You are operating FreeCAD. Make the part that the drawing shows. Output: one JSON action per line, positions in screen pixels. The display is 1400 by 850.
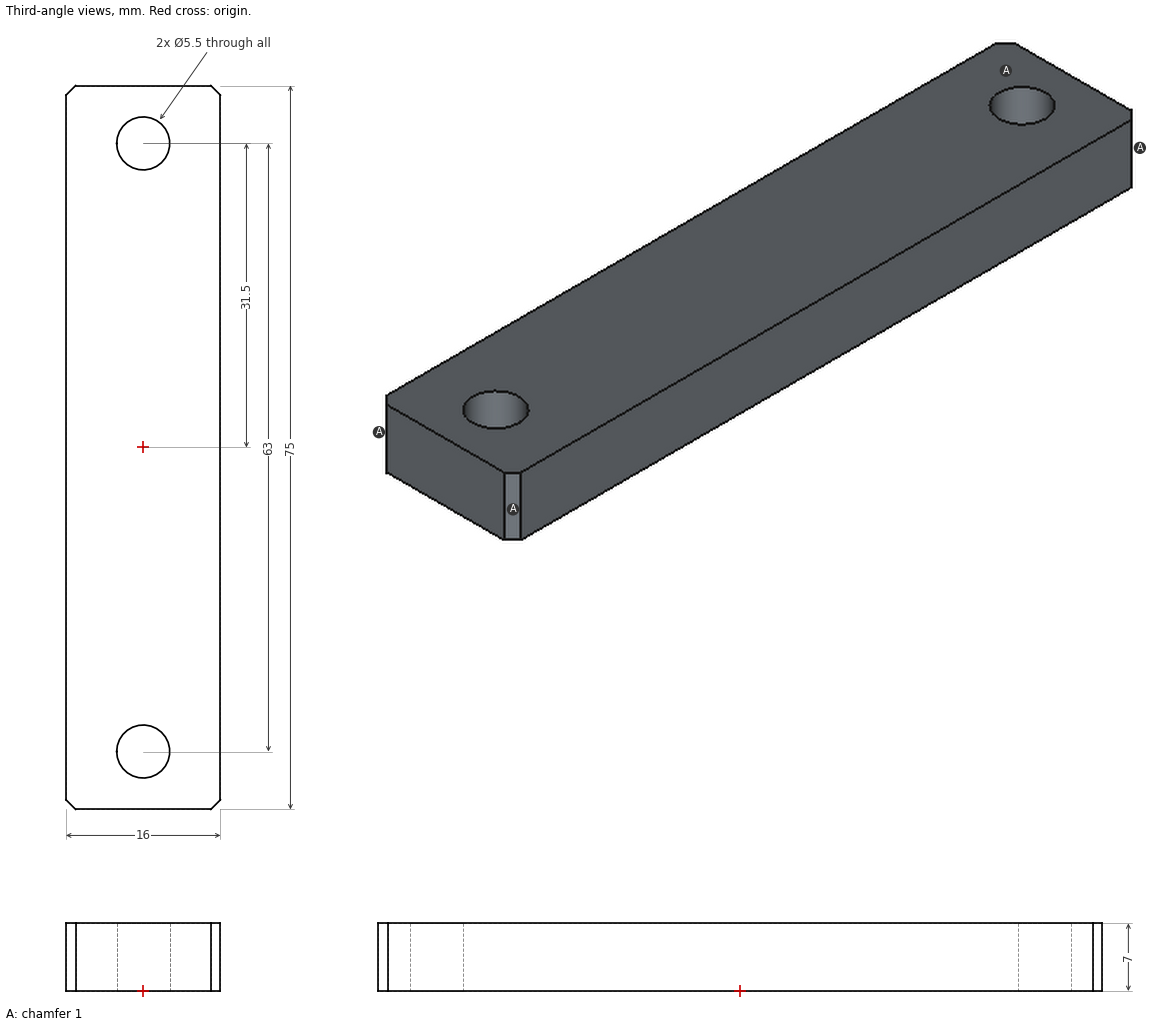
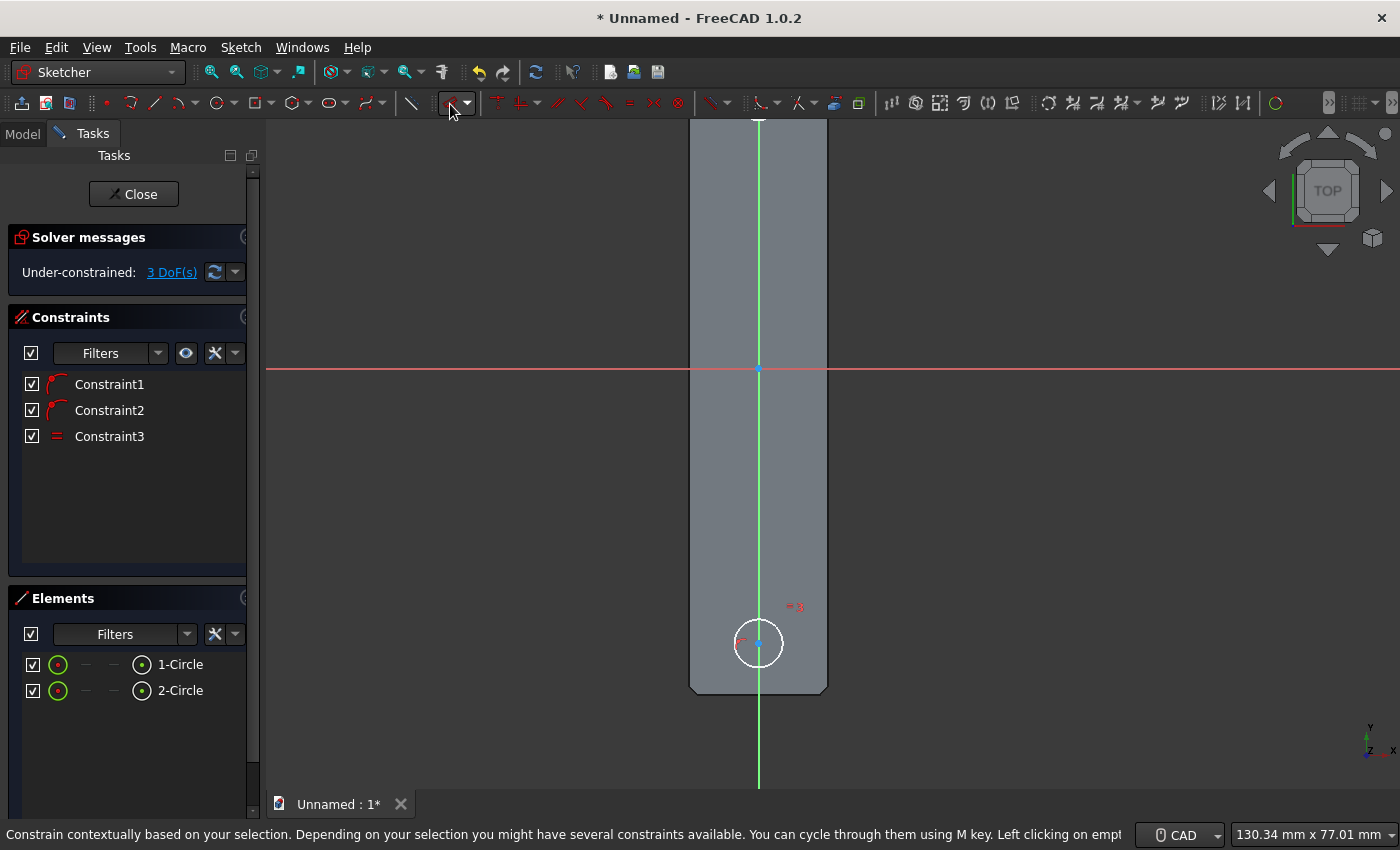
{"action": "scroll", "coordinate": [776, 627], "scroll_direction": "down", "scroll_amount": 2}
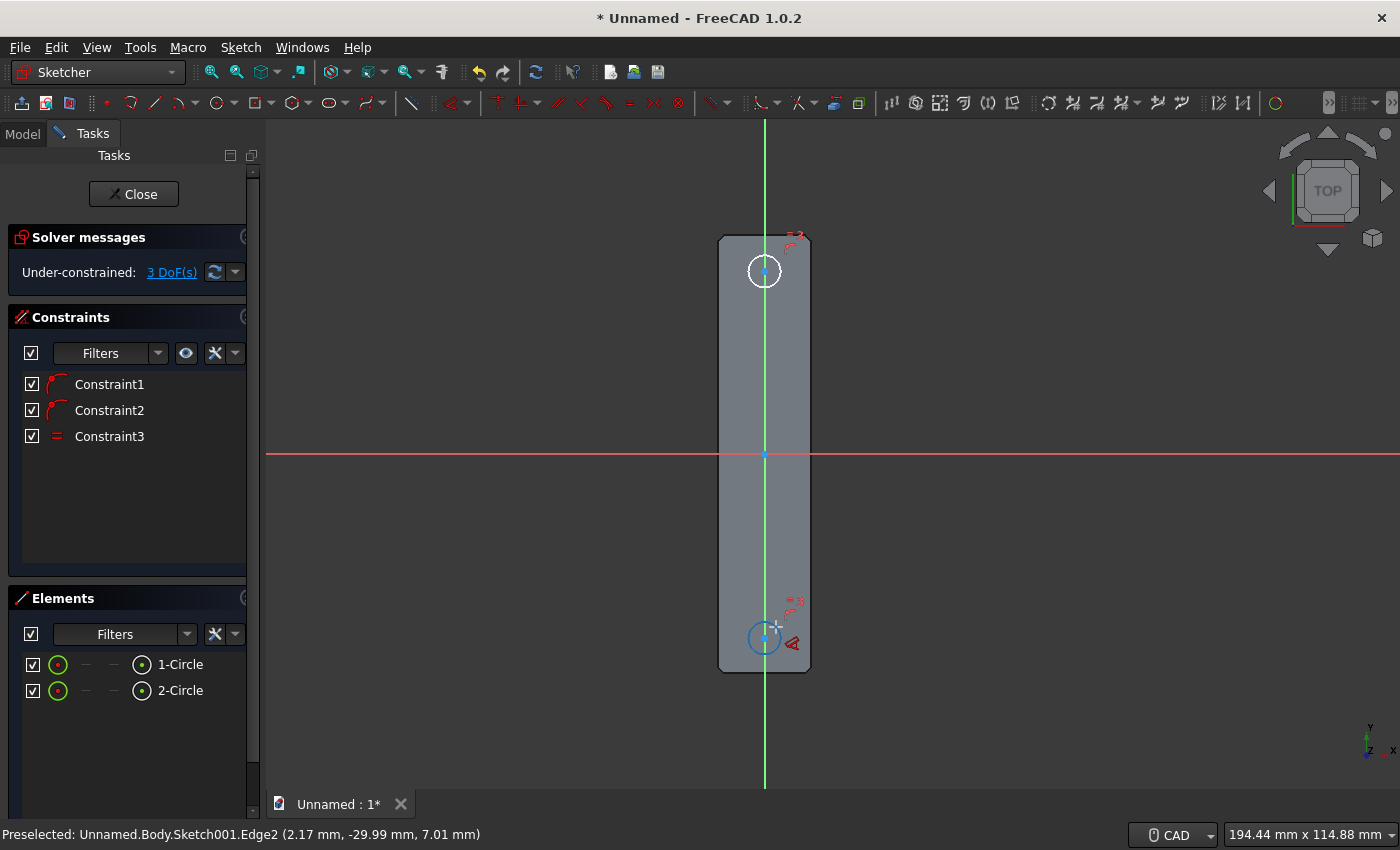
{"action": "scroll", "coordinate": [776, 260], "scroll_direction": "up", "scroll_amount": 2}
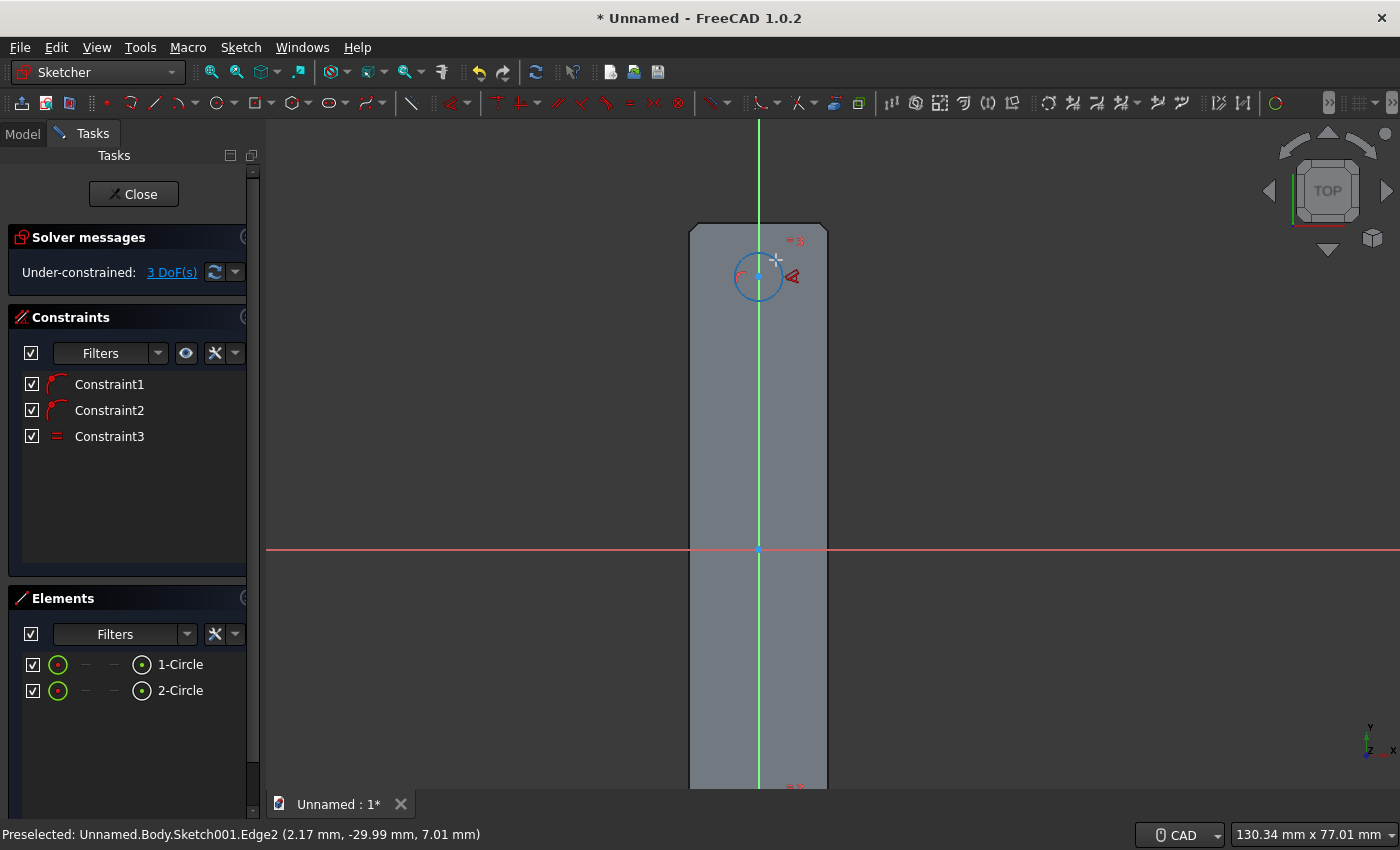
{"action": "left_click", "coordinate": [776, 260]}
{"action": "left_click", "coordinate": [799, 238]}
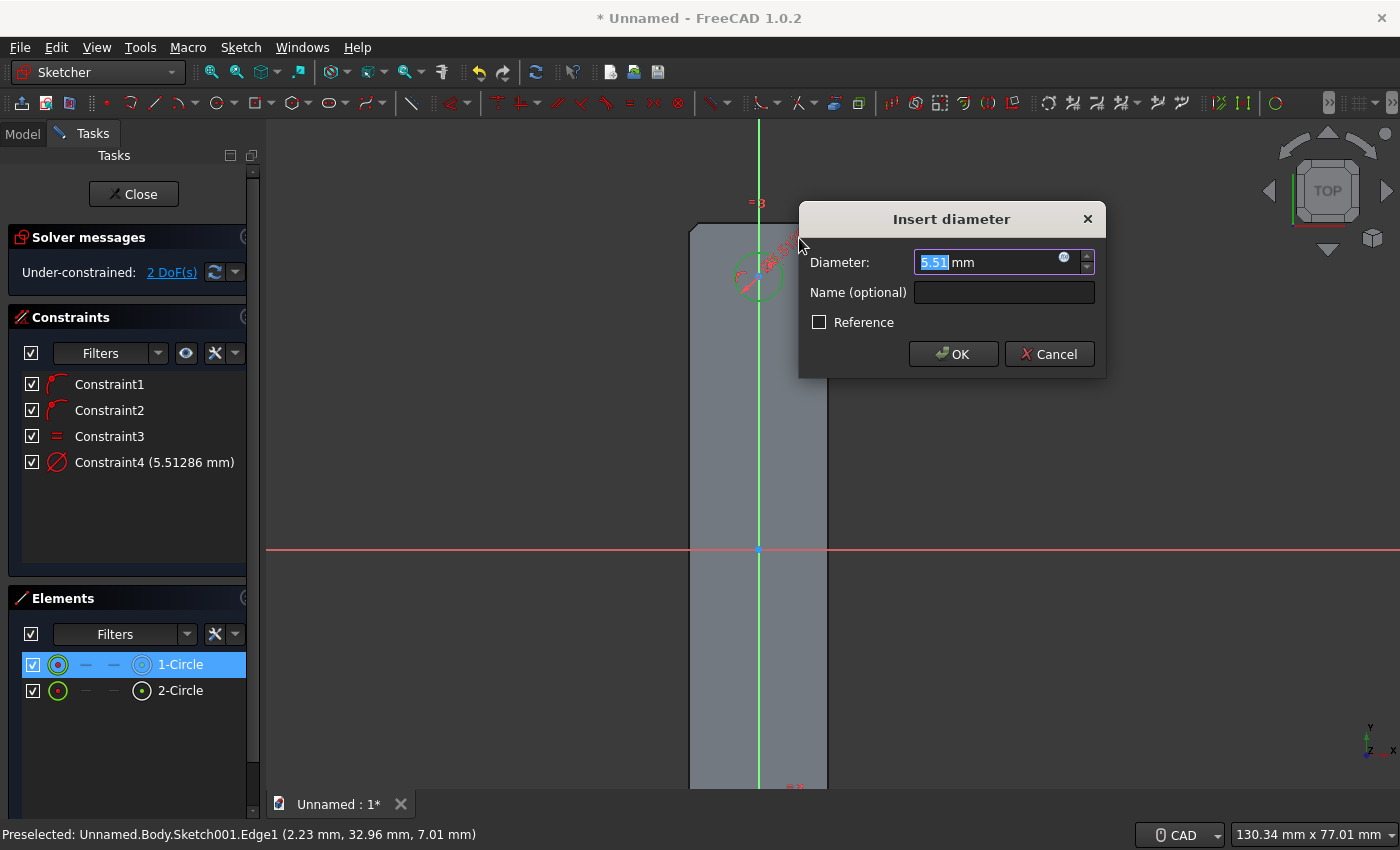
{"action": "type", "text": "5.5"}
{"action": "key", "text": "Return"}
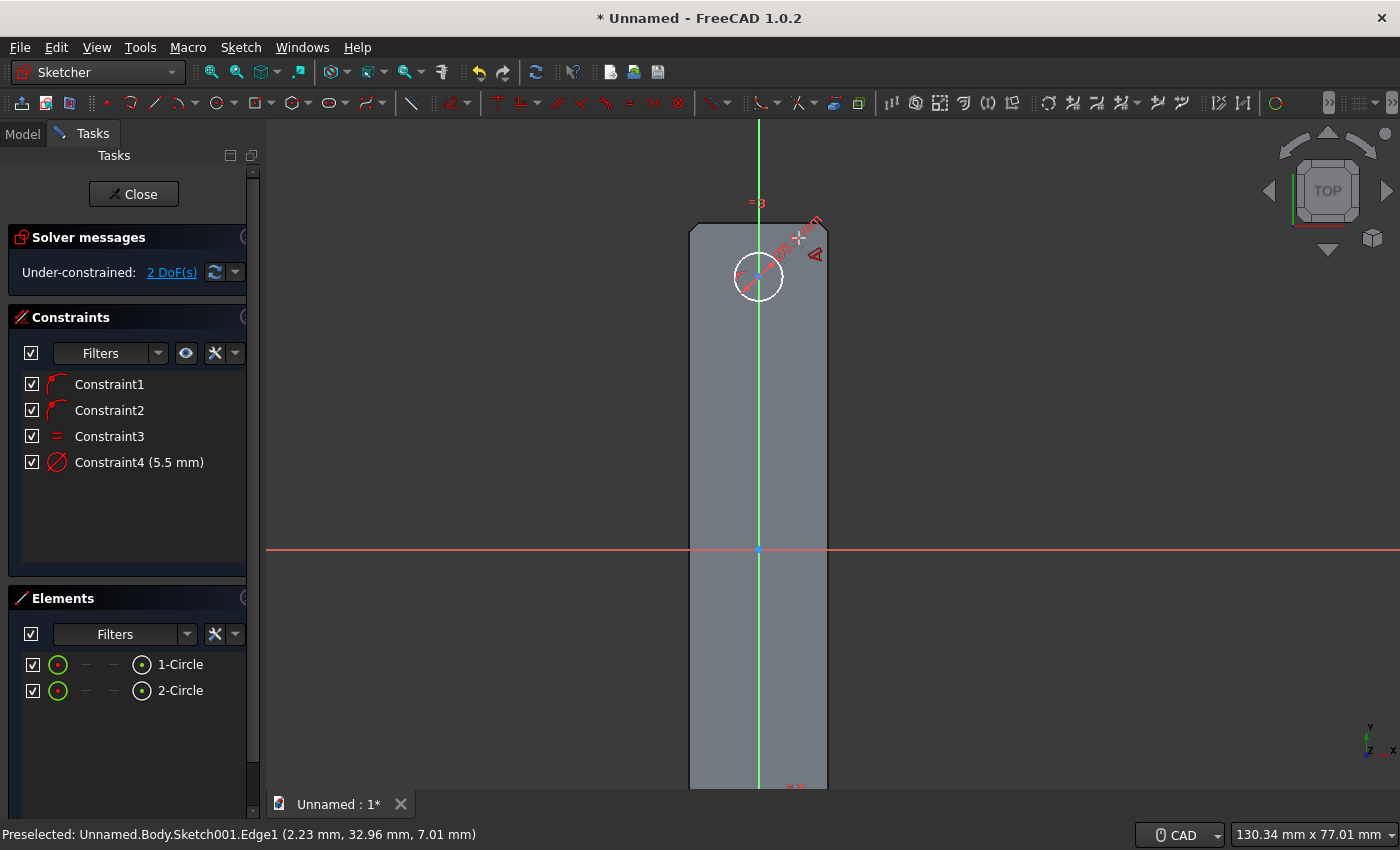
{"action": "left_click", "coordinate": [759, 277]}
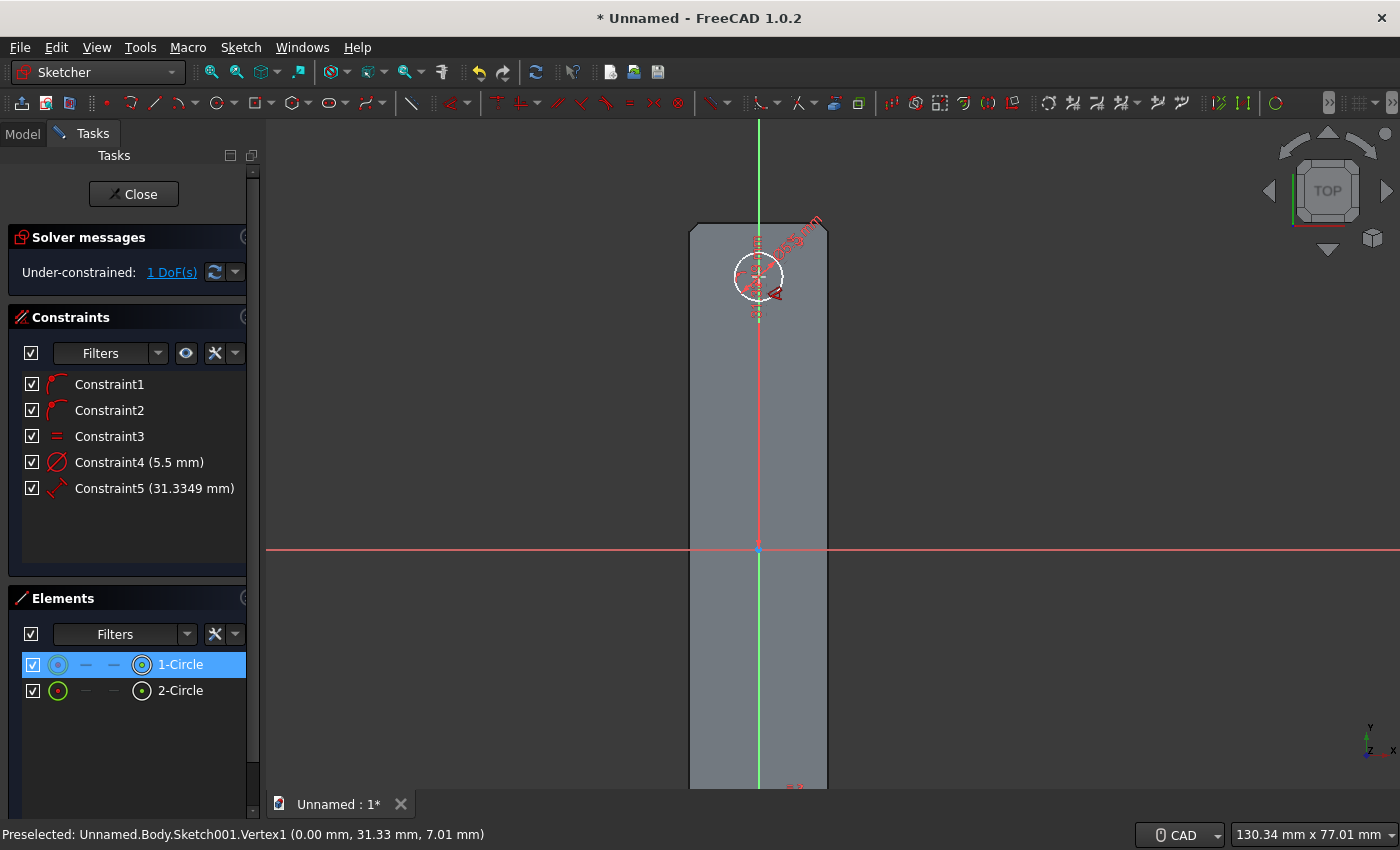
{"action": "scroll", "coordinate": [776, 260], "scroll_direction": "down", "scroll_amount": 2}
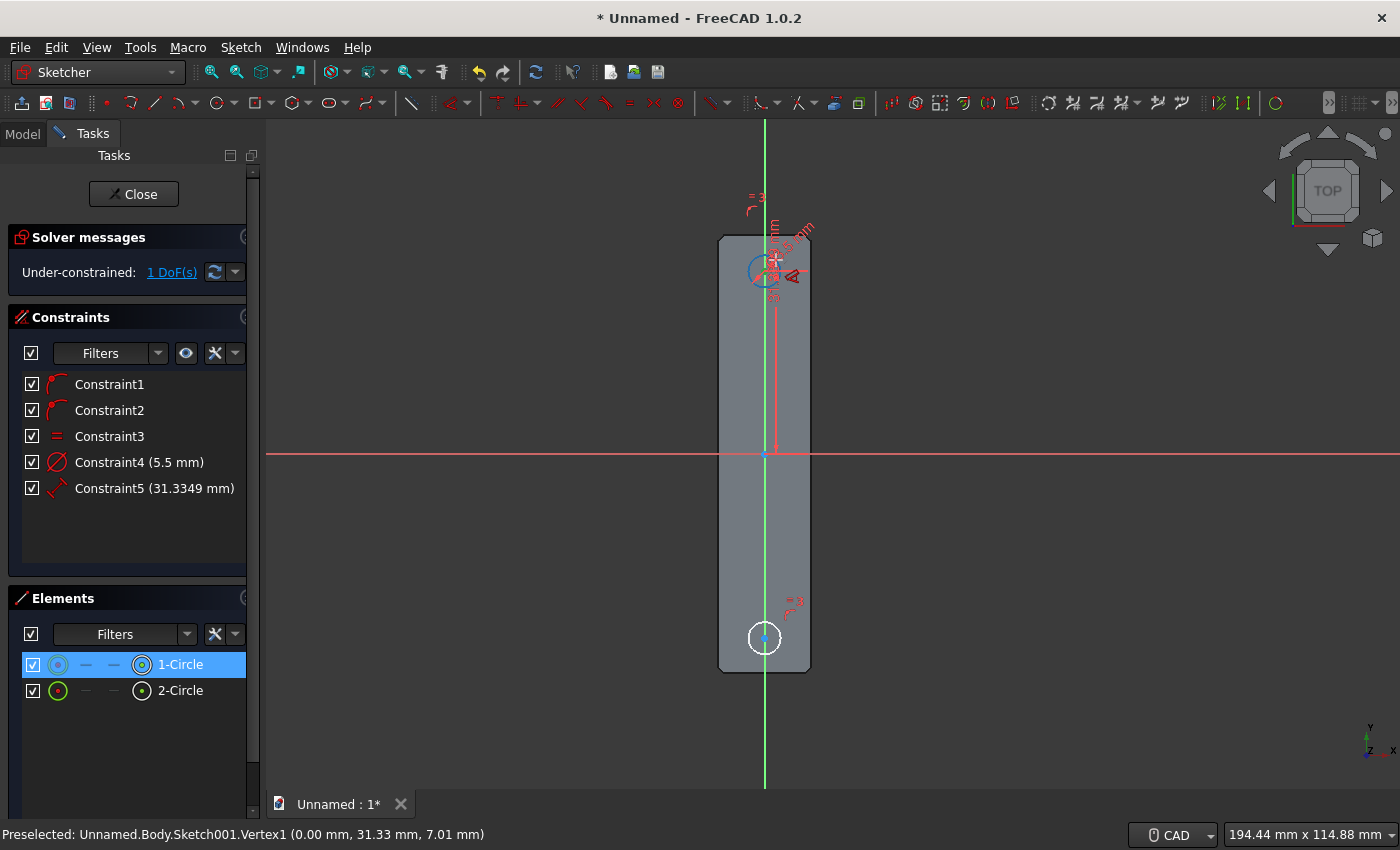
{"action": "left_click", "coordinate": [765, 638]}
{"action": "left_click", "coordinate": [799, 370]}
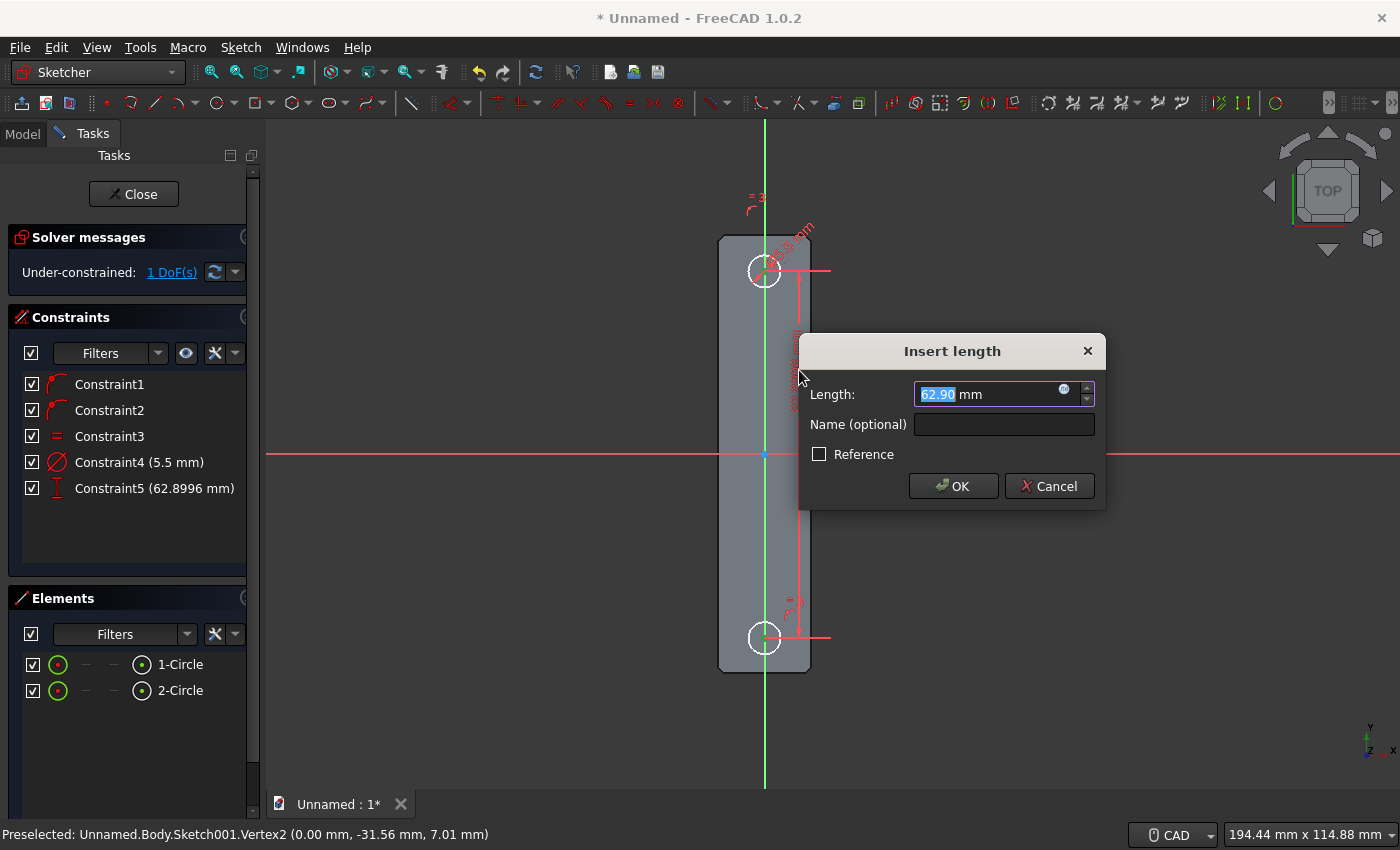
{"action": "type", "text": "63"}
{"action": "key", "text": "Return"}